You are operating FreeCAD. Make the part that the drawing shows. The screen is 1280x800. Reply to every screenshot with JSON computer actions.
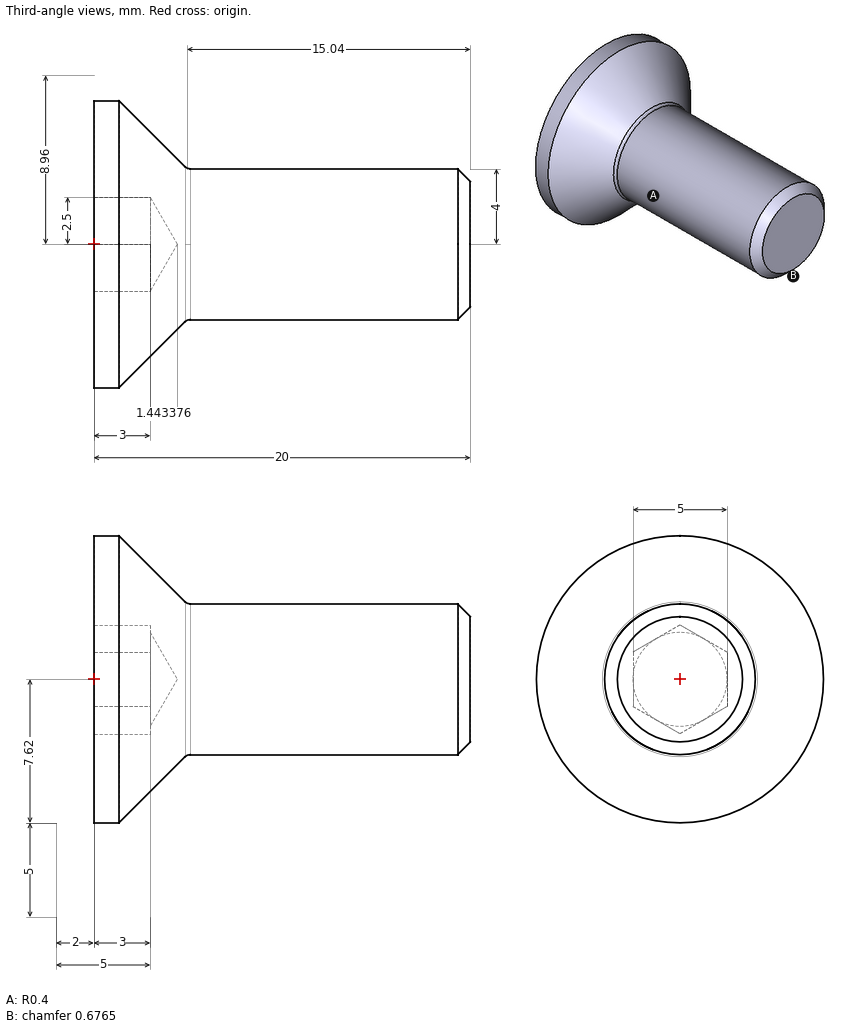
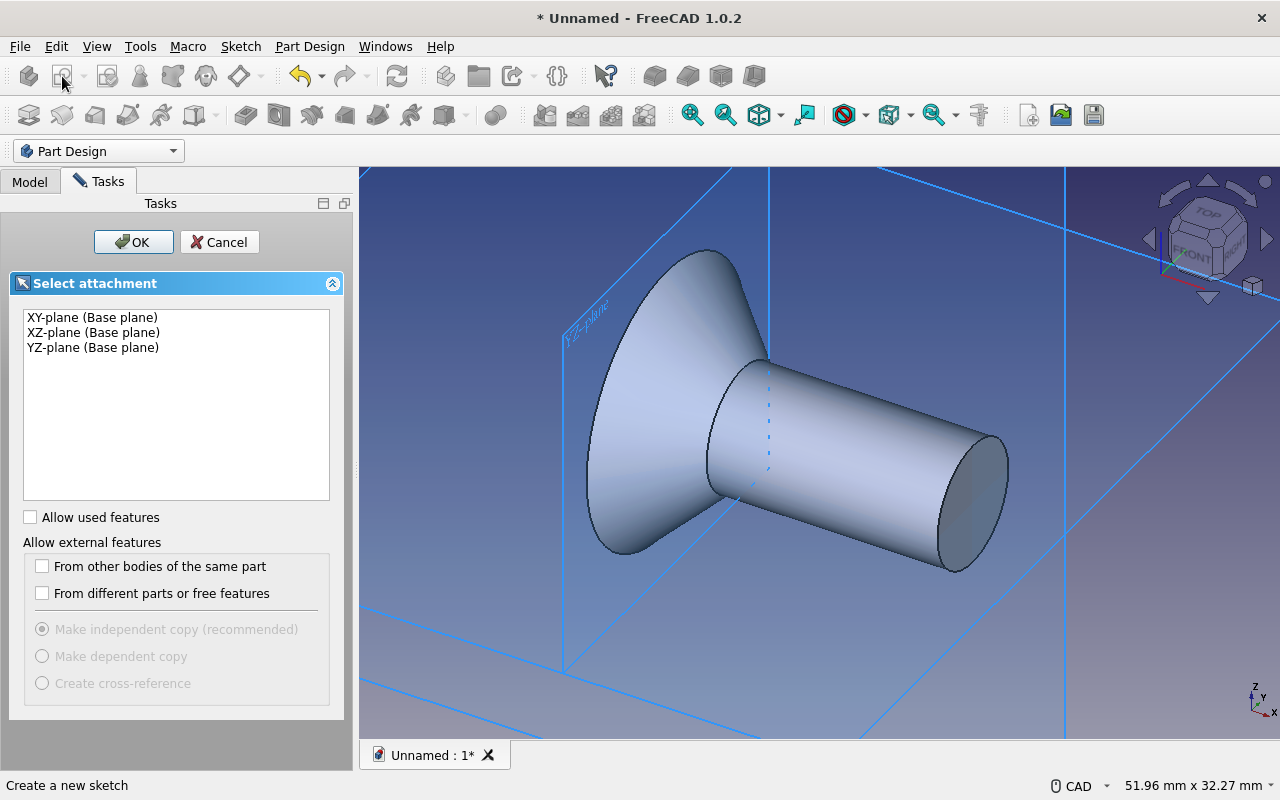
{"action": "left_click", "coordinate": [84, 318]}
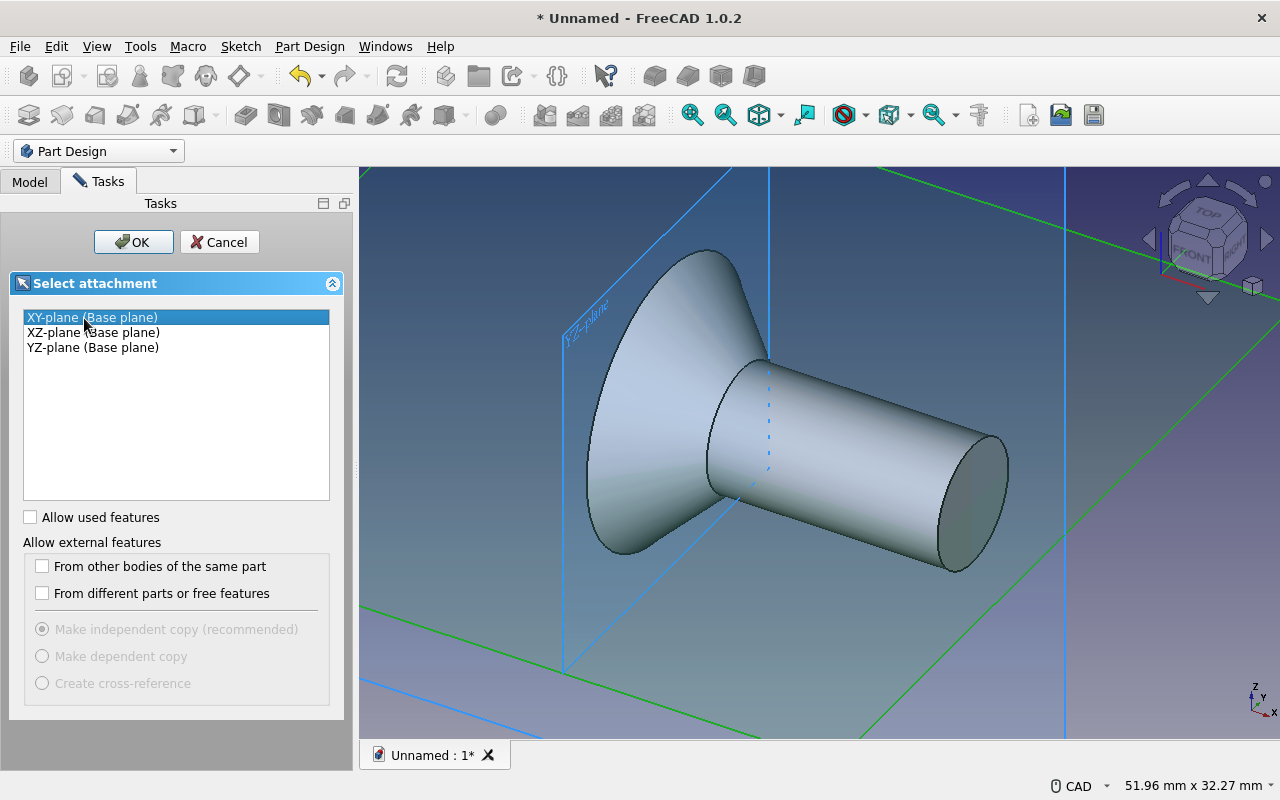
{"action": "left_click", "coordinate": [134, 242]}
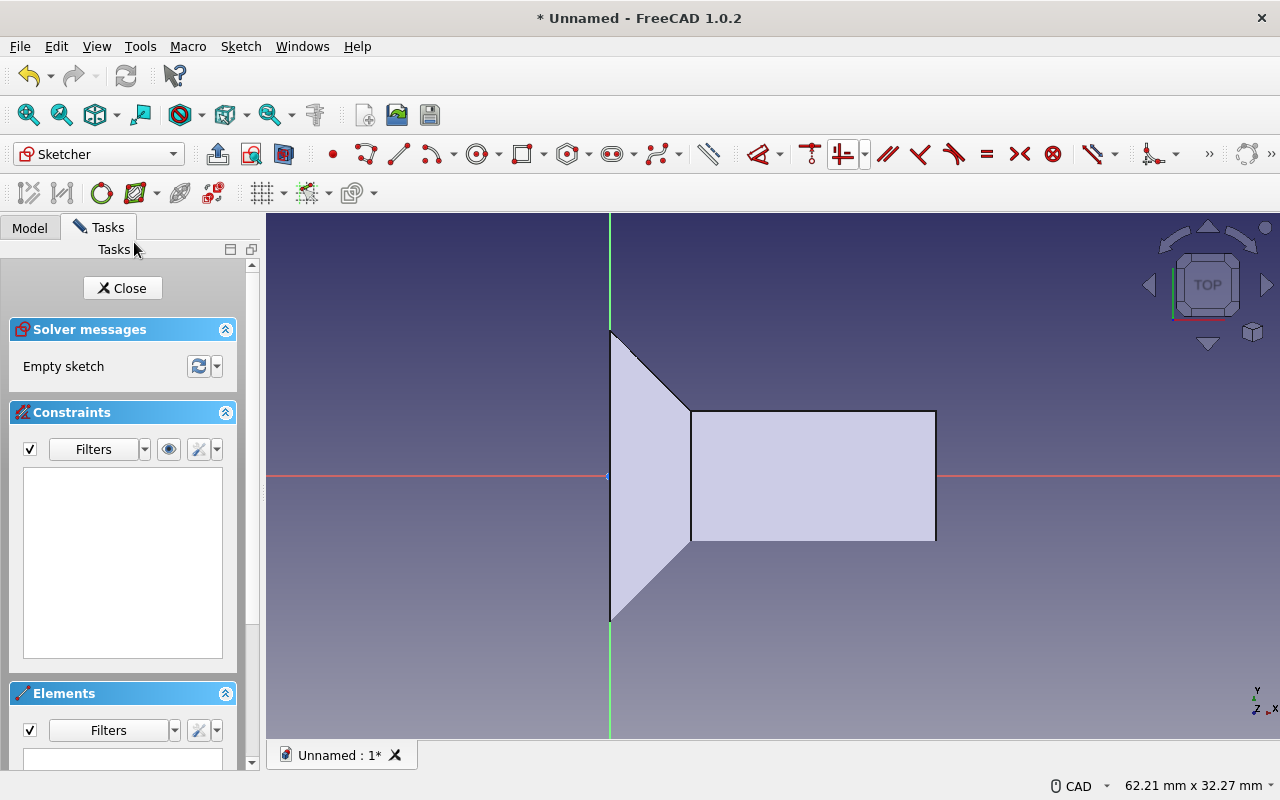
{"action": "left_click", "coordinate": [284, 154]}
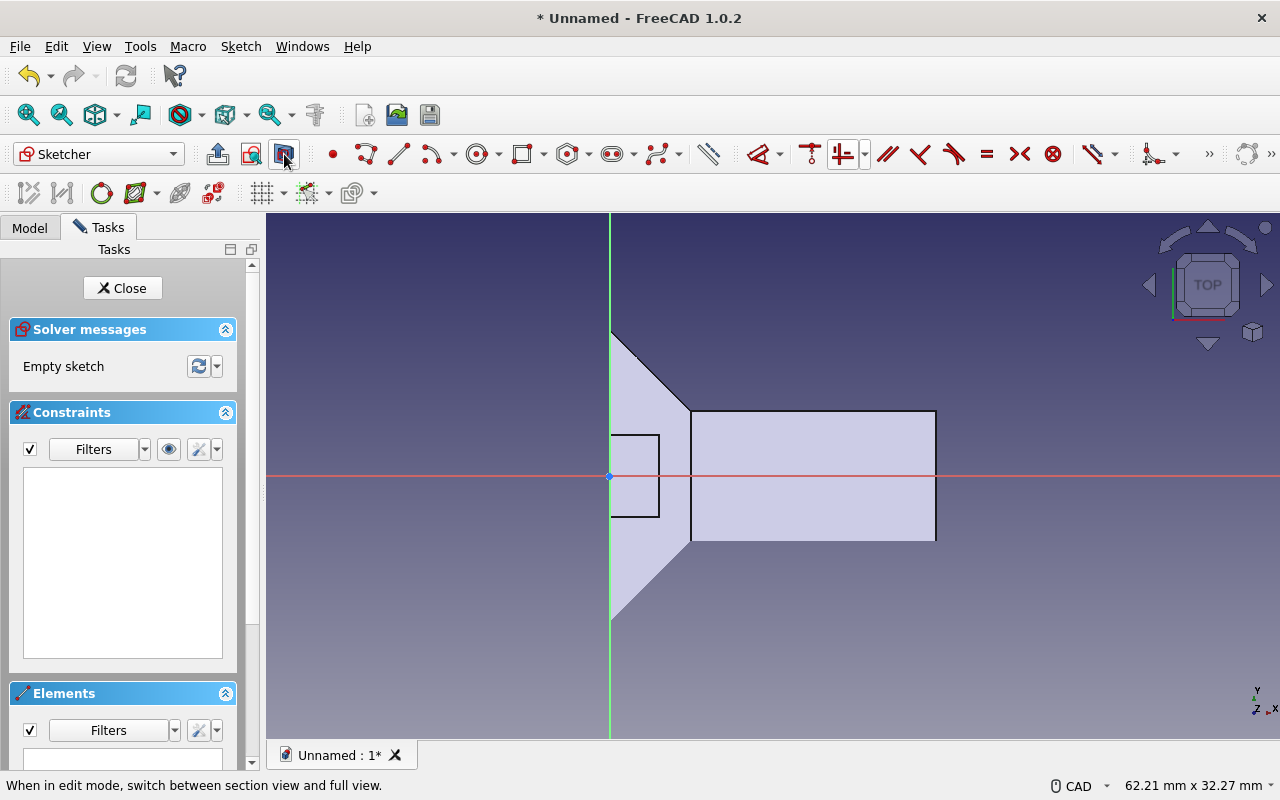
{"action": "scroll", "coordinate": [637, 453], "scroll_direction": "up", "scroll_amount": 10}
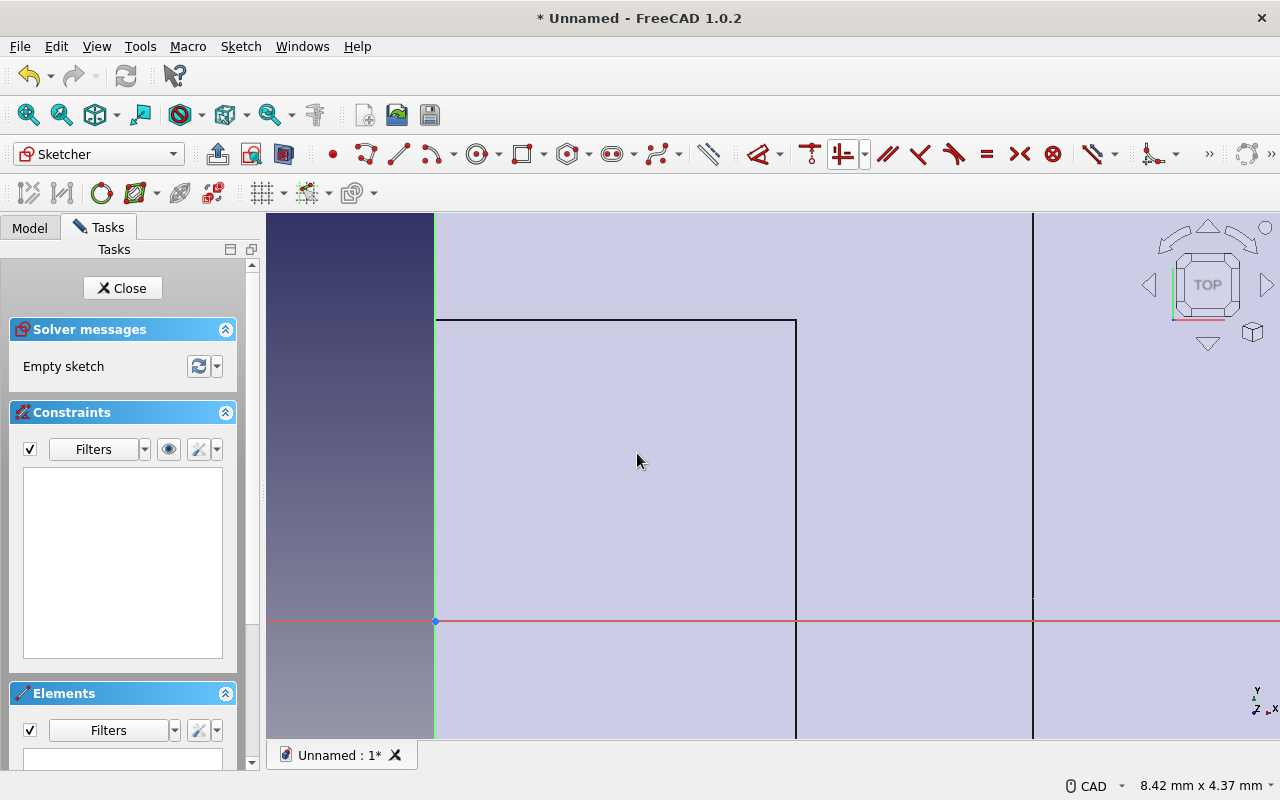
{"action": "left_click", "coordinate": [366, 154]}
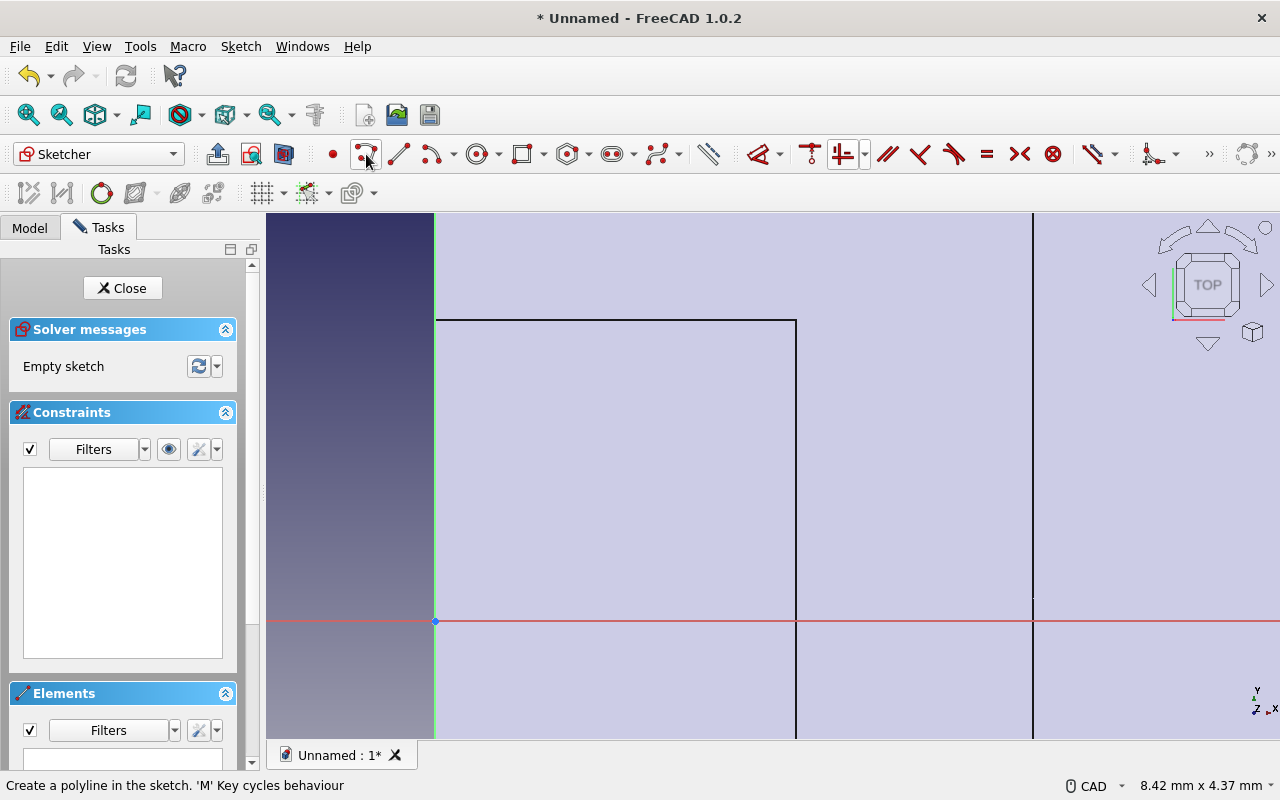
{"action": "left_click", "coordinate": [796, 621]}
{"action": "left_click", "coordinate": [970, 612]}
{"action": "left_click", "coordinate": [796, 320]}
{"action": "left_click", "coordinate": [796, 621]}
{"action": "key", "text": "Escape"}
{"action": "key", "text": "Escape"}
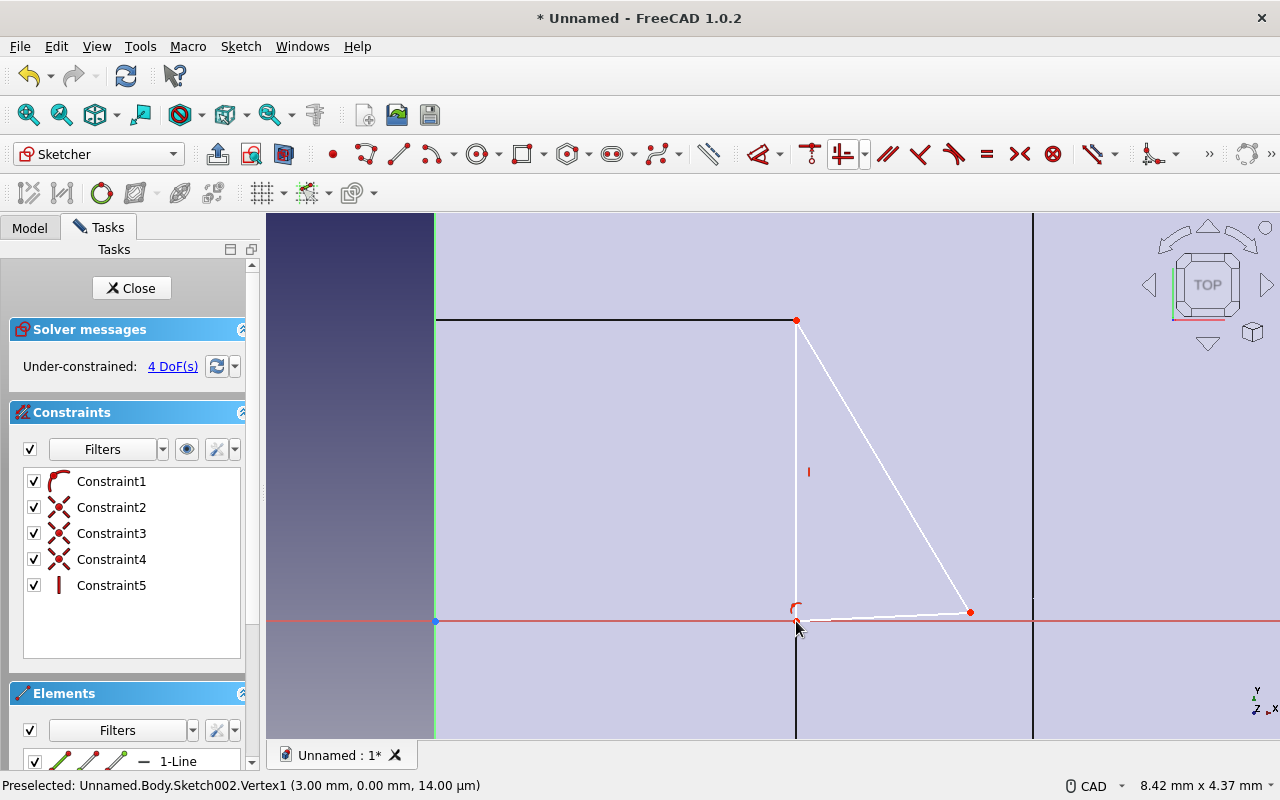
{"action": "left_click", "coordinate": [848, 619]}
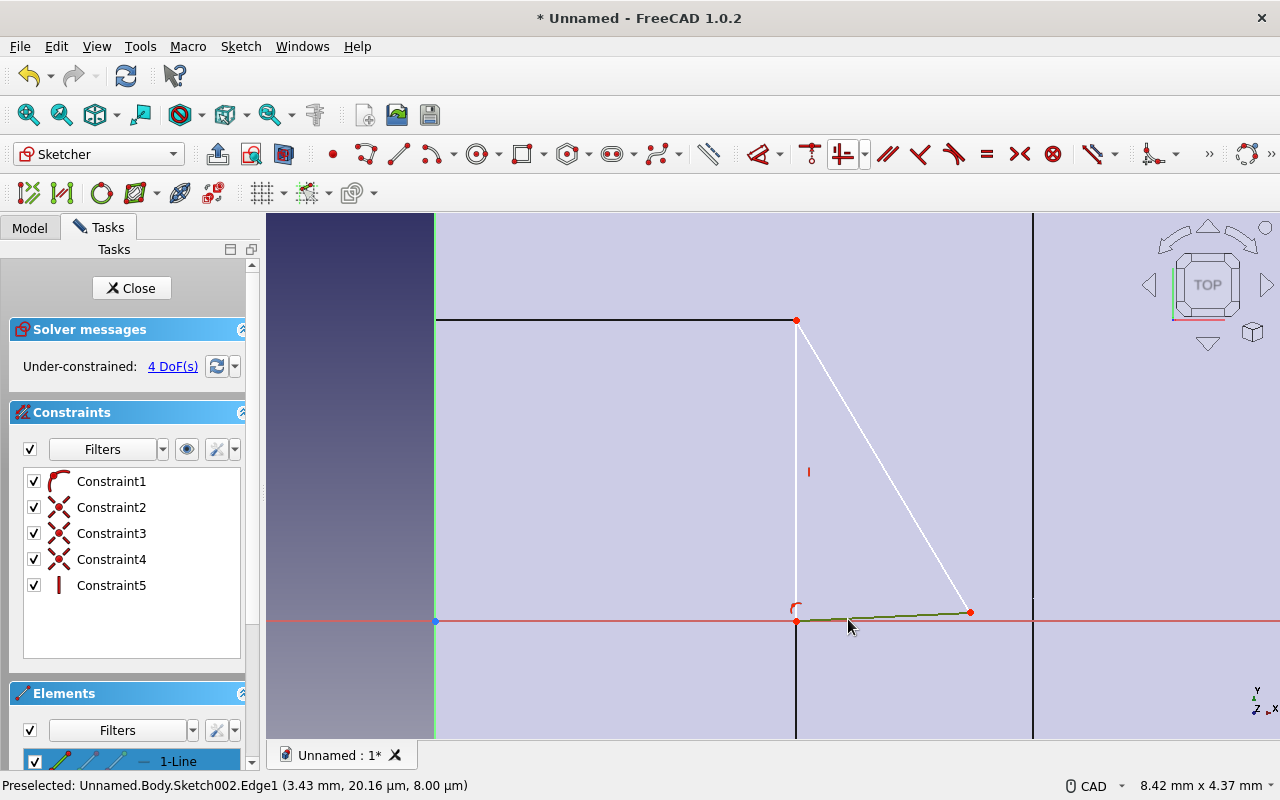
{"action": "key", "text": "h"}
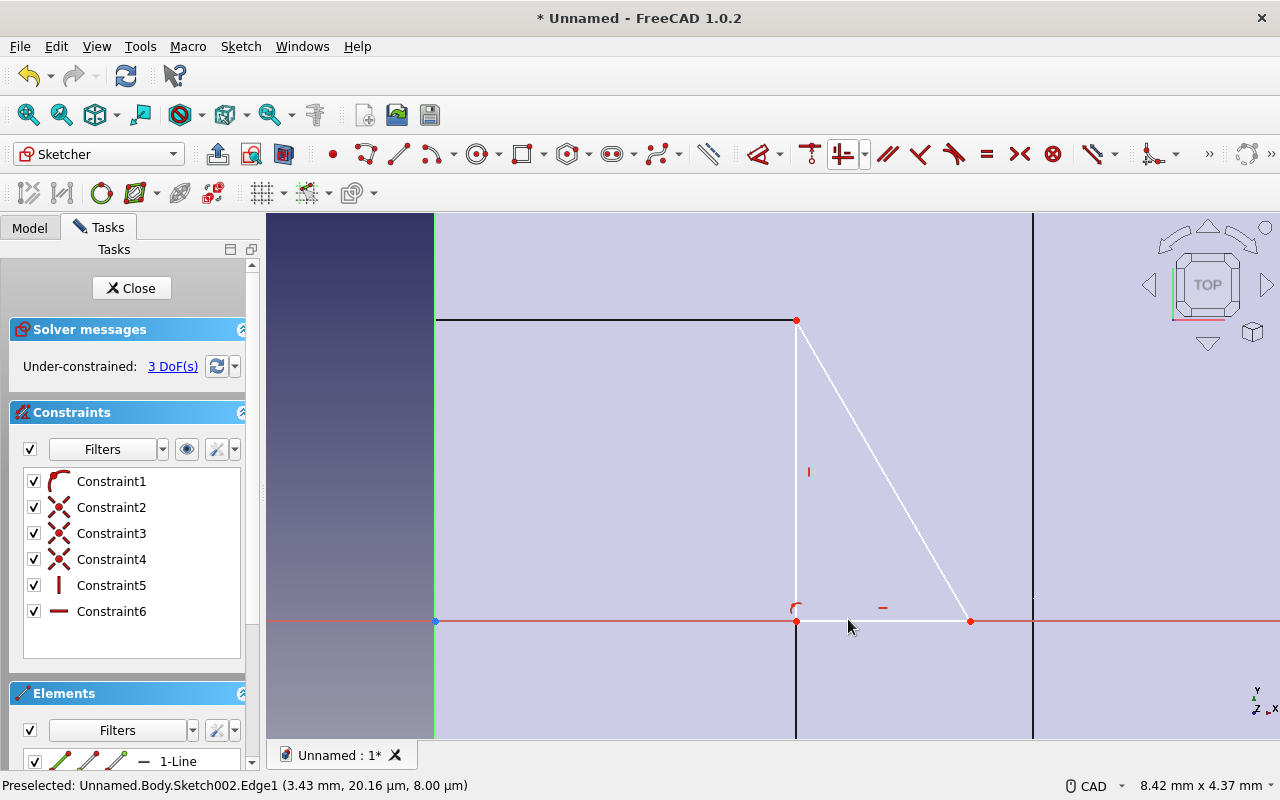
{"action": "left_click", "coordinate": [758, 154]}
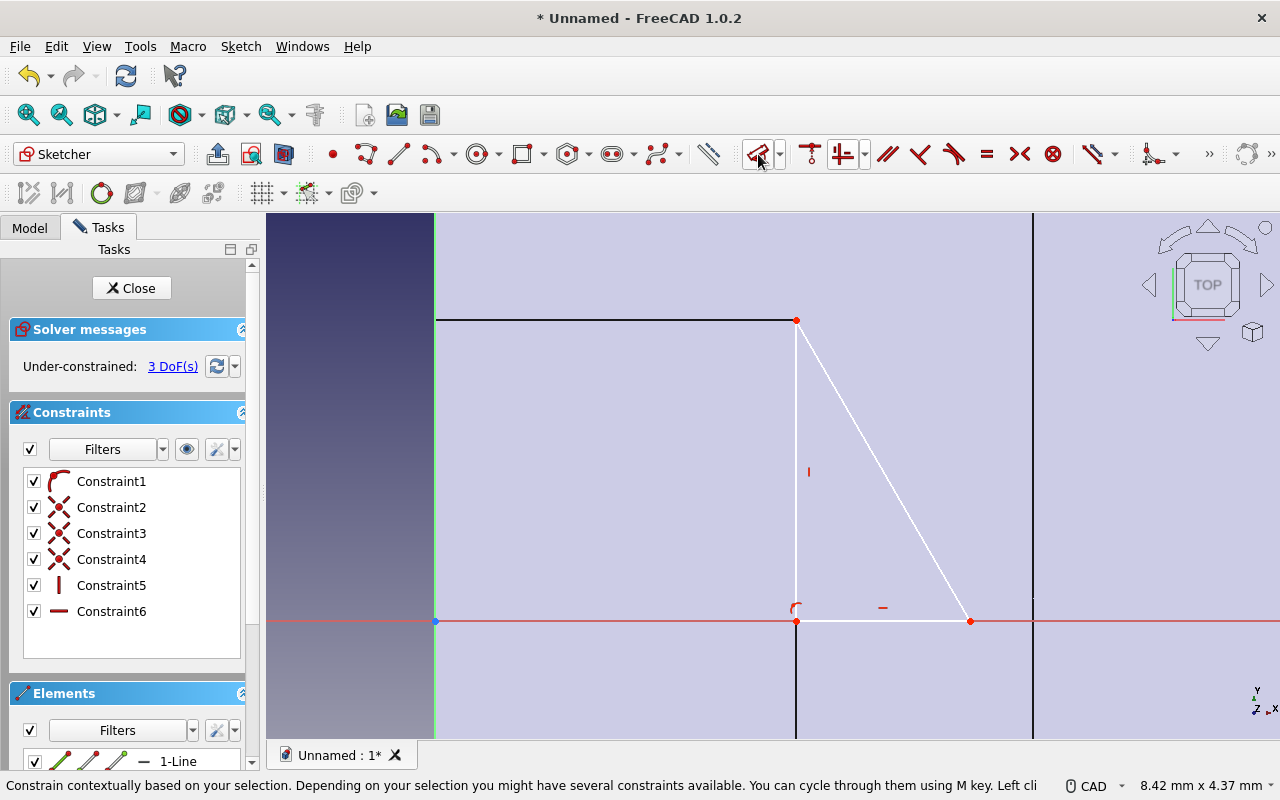
{"action": "left_click", "coordinate": [796, 621]}
{"action": "left_click", "coordinate": [616, 655]}